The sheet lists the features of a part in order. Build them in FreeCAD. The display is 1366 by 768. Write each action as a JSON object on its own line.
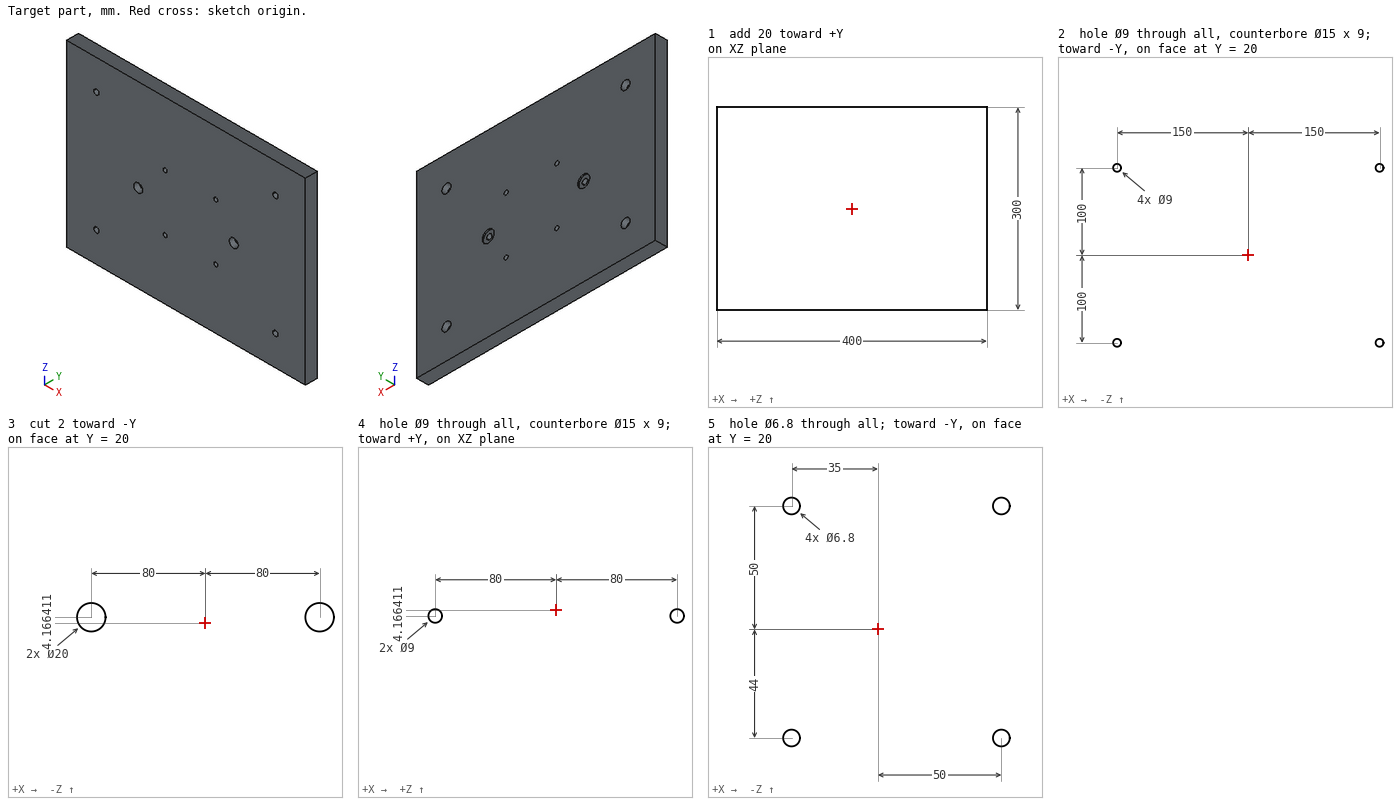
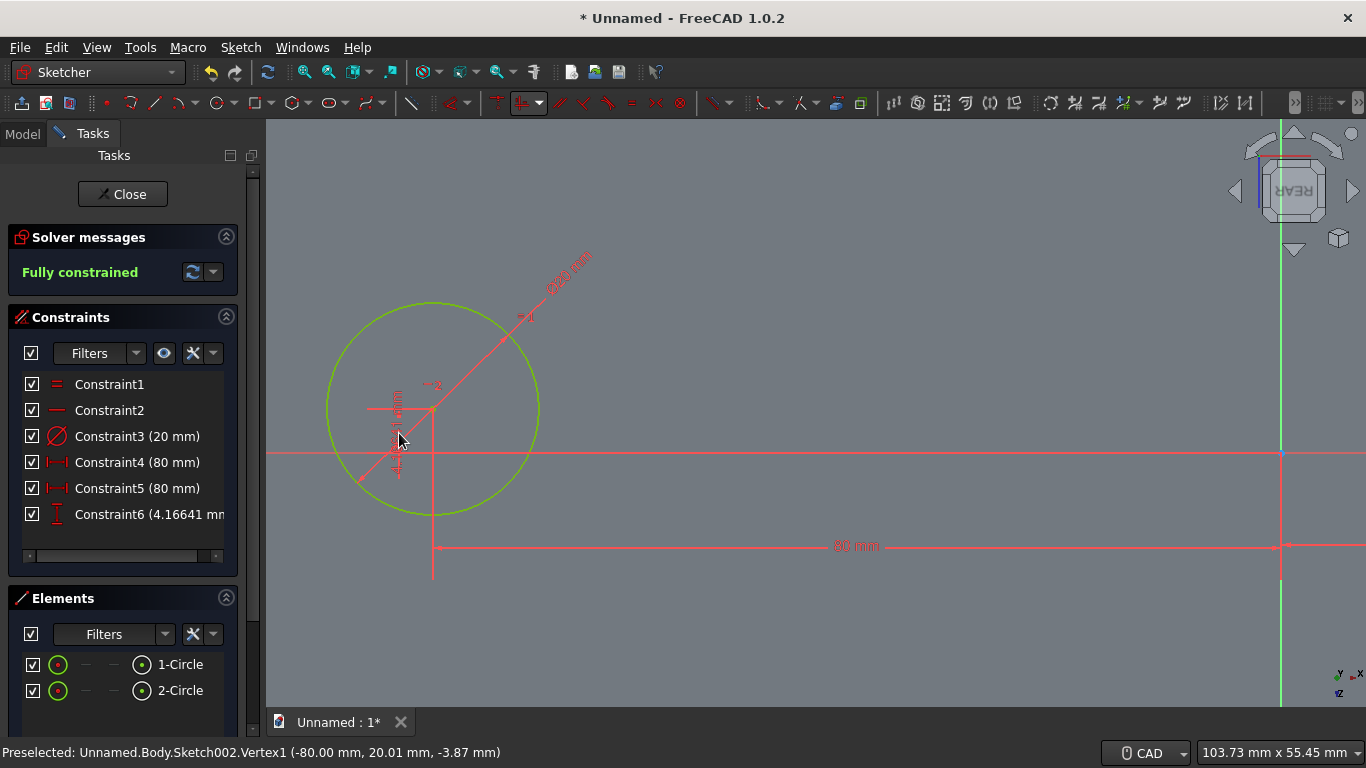
{"action": "left_click", "coordinate": [123, 194]}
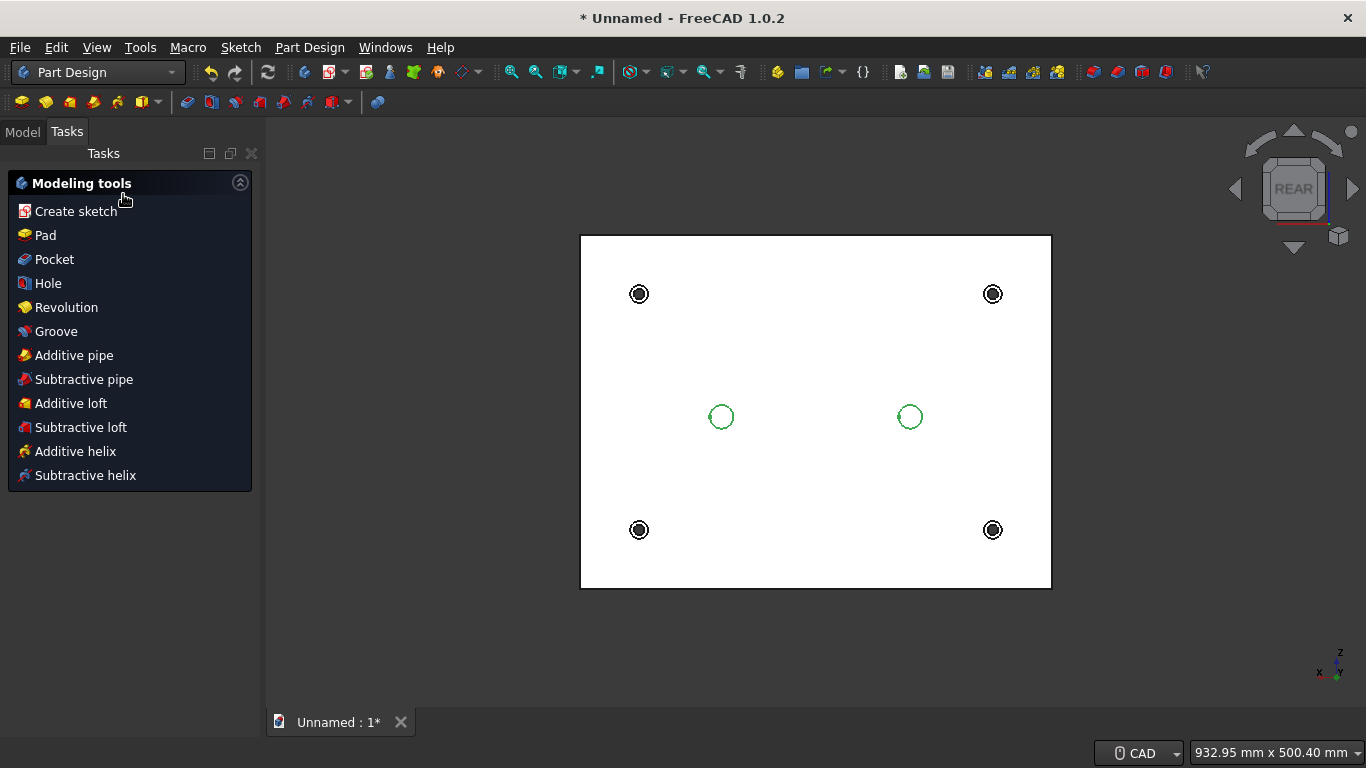
{"action": "left_click", "coordinate": [188, 102]}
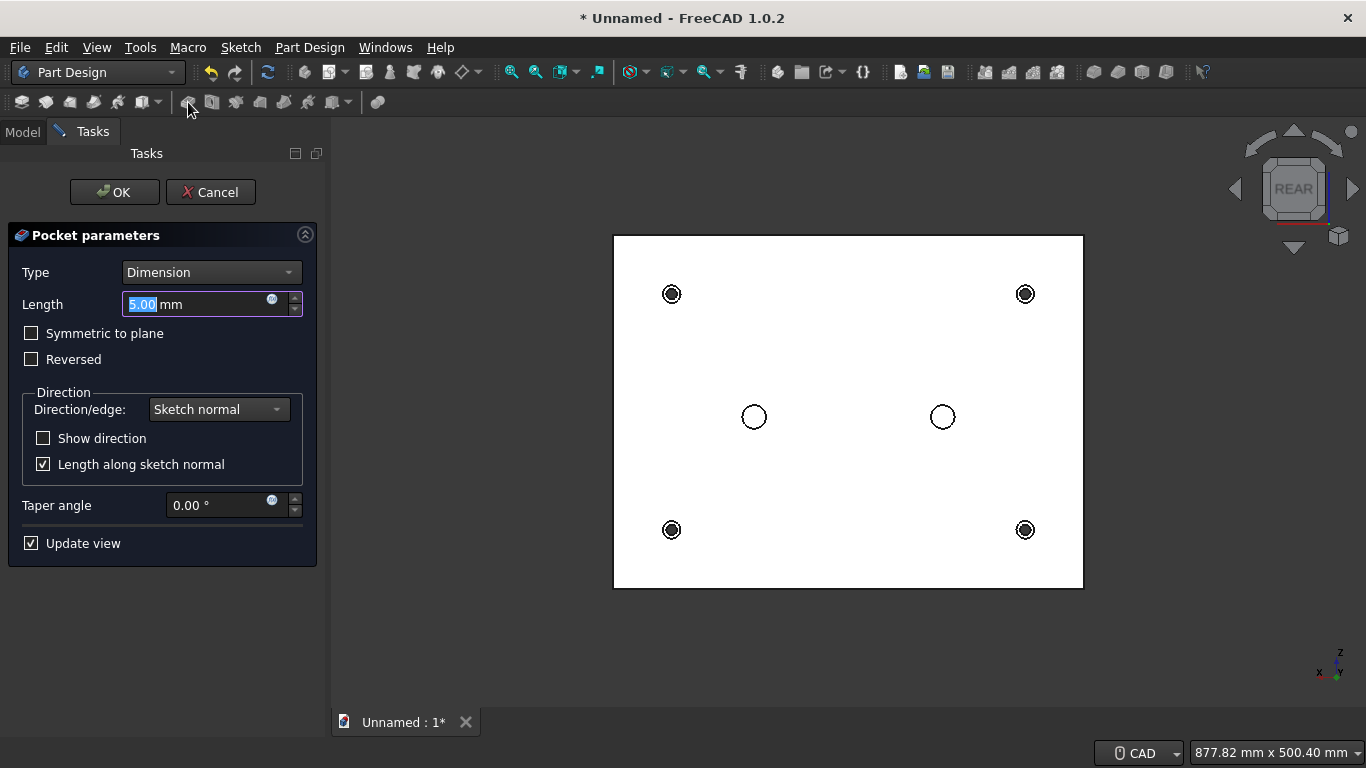
{"action": "type", "text": "2"}
{"action": "key", "text": "Tab"}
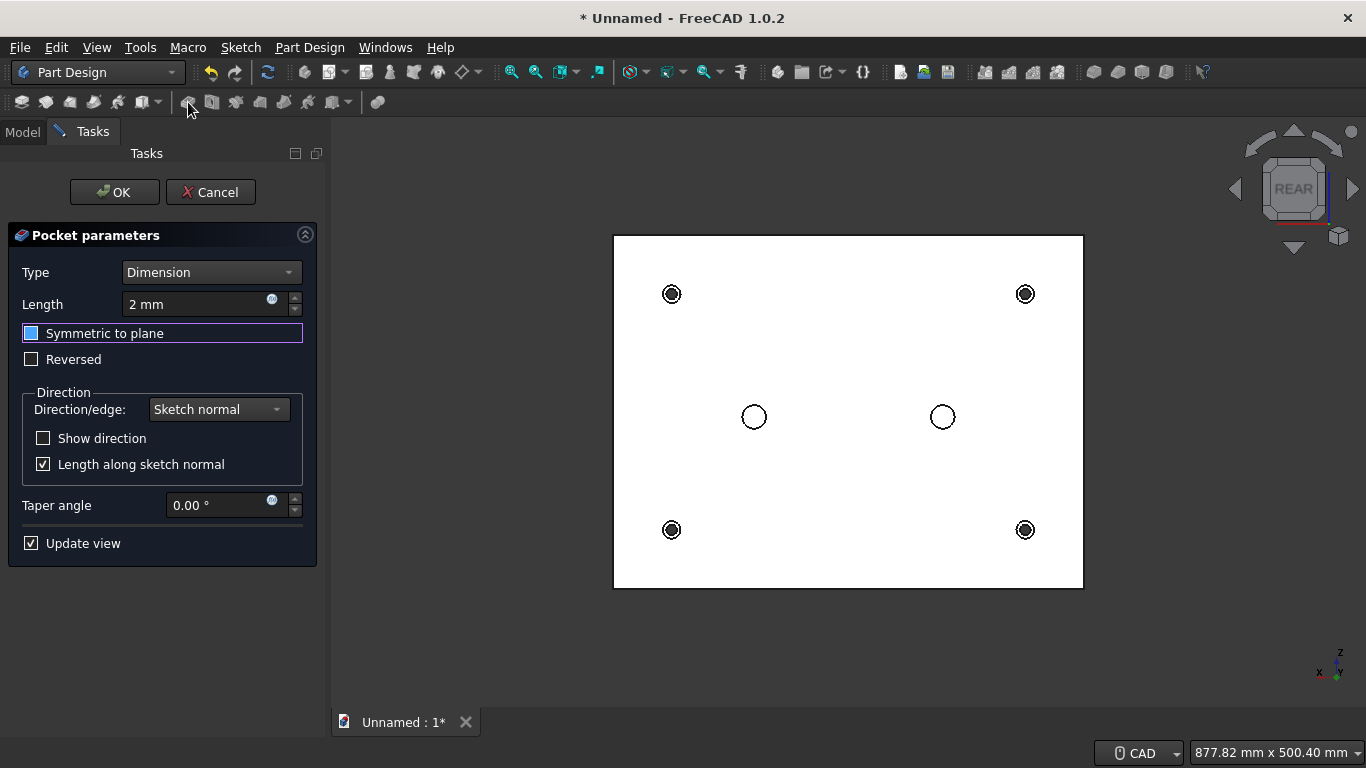
{"action": "left_click", "coordinate": [115, 192]}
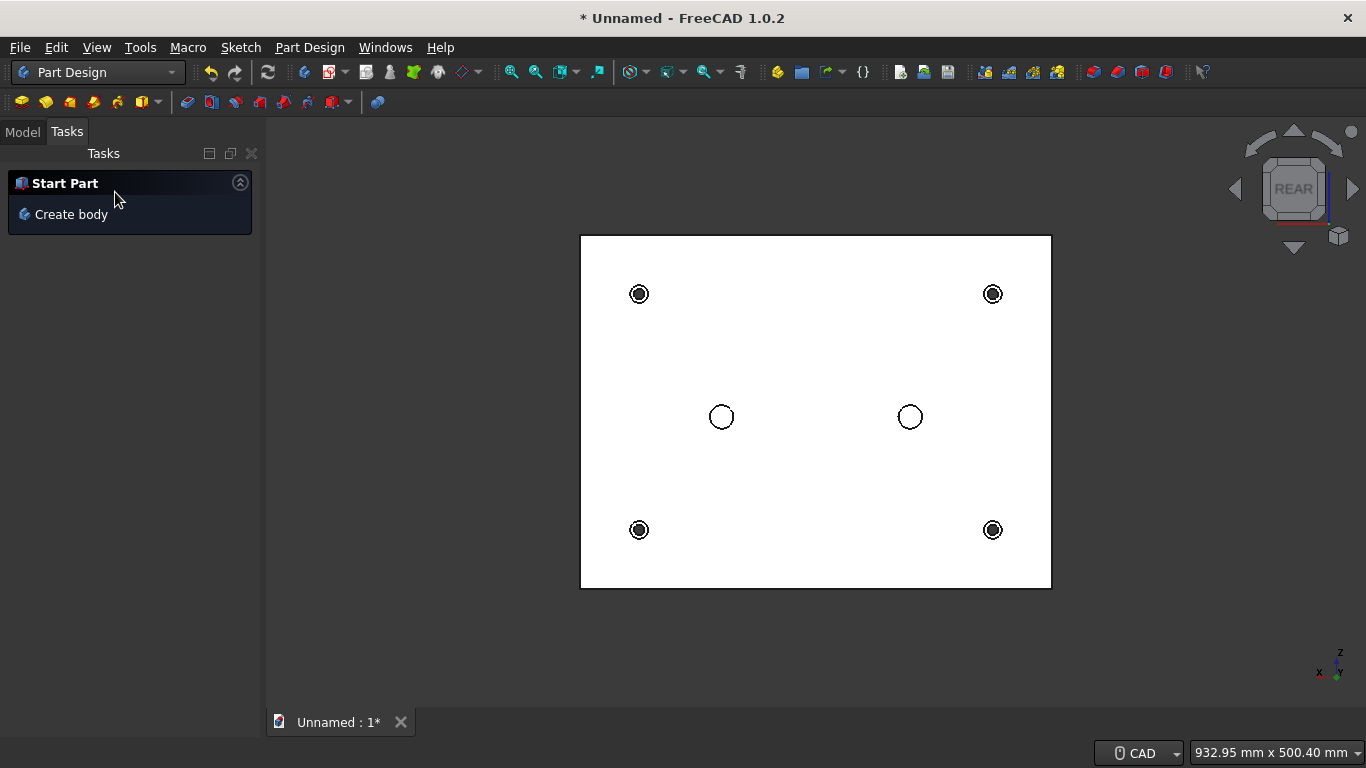
{"action": "left_click", "coordinate": [330, 72]}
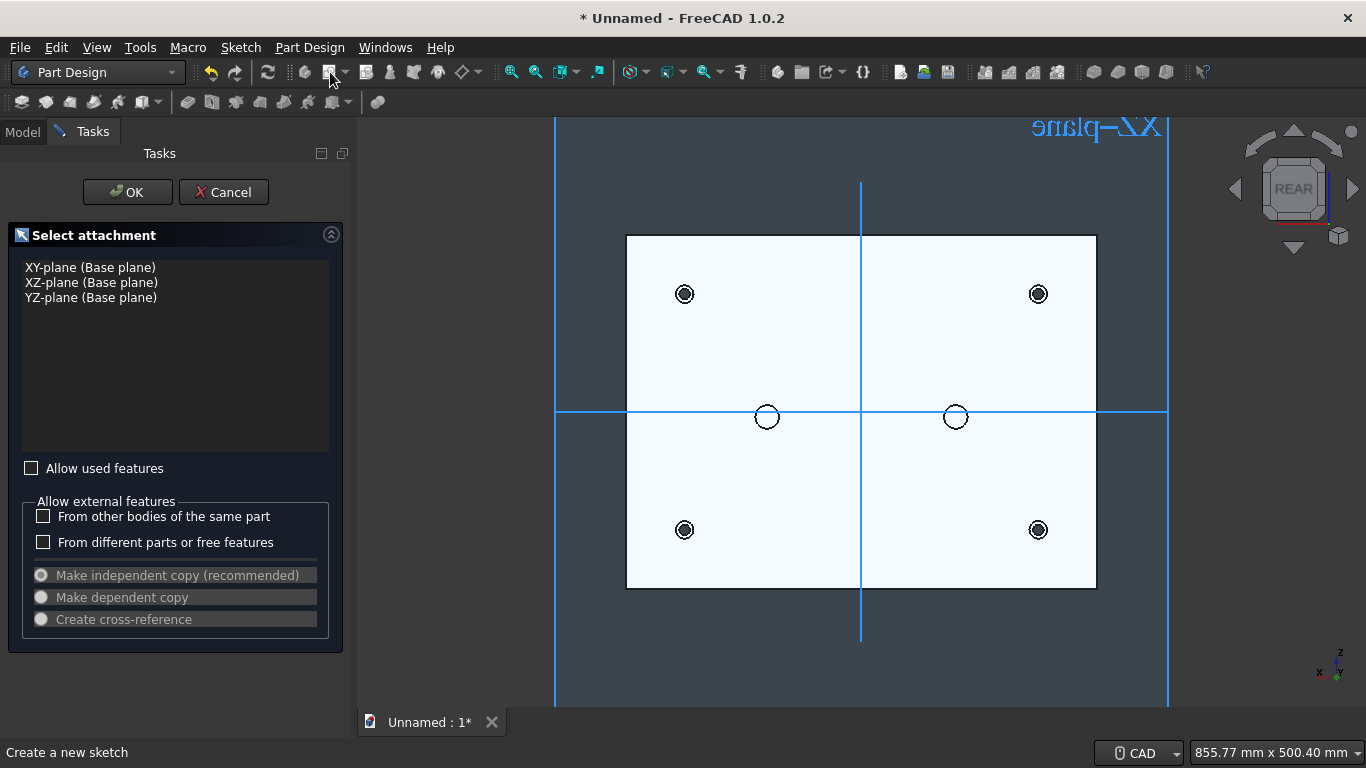
{"action": "left_click", "coordinate": [82, 282]}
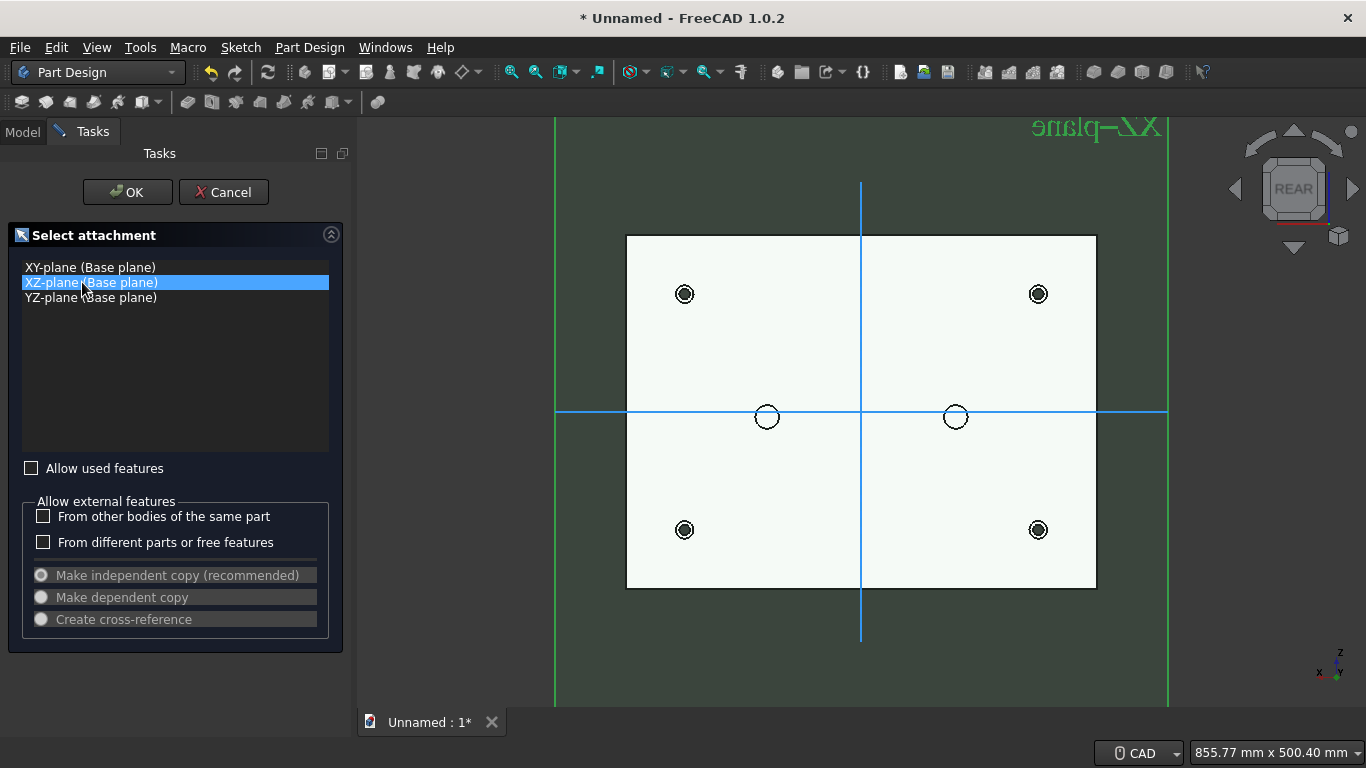
{"action": "left_click", "coordinate": [128, 192]}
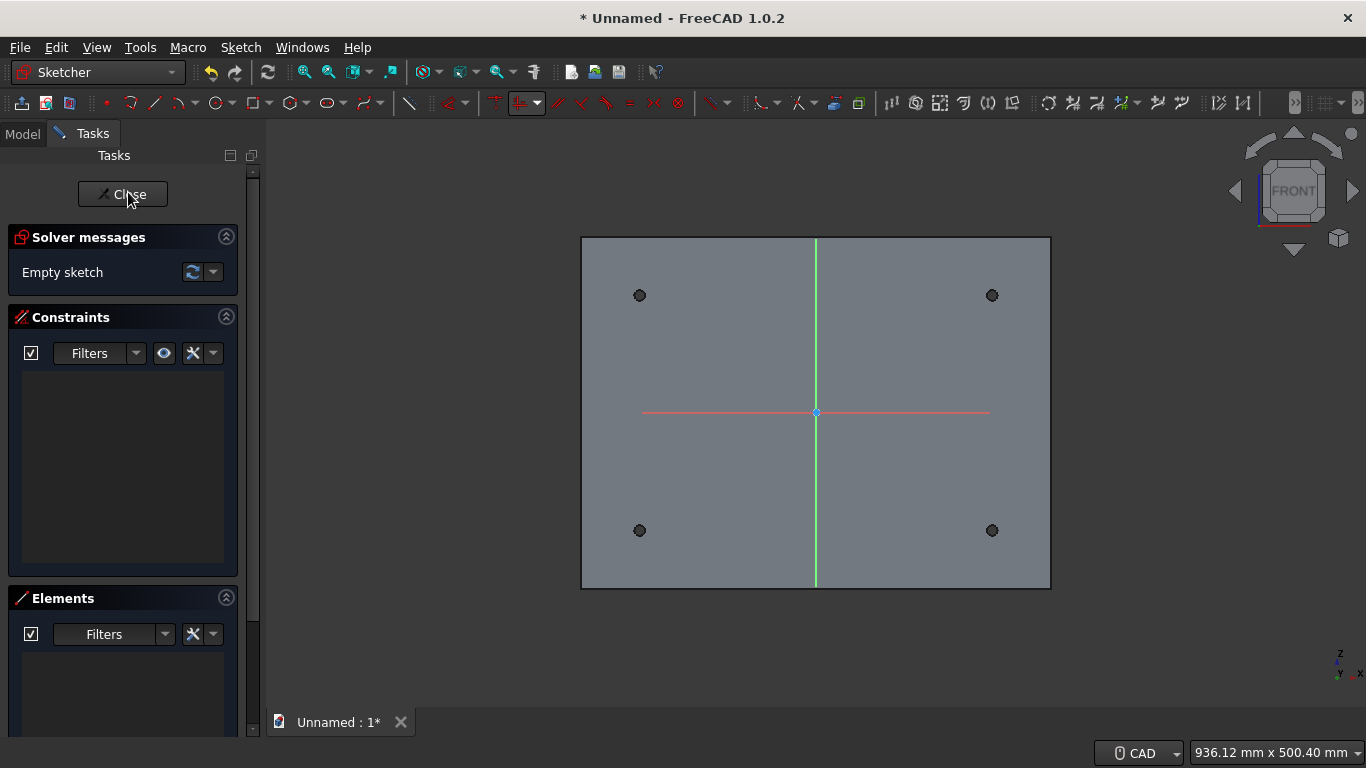
{"action": "scroll", "coordinate": [846, 420], "scroll_direction": "up", "scroll_amount": 6}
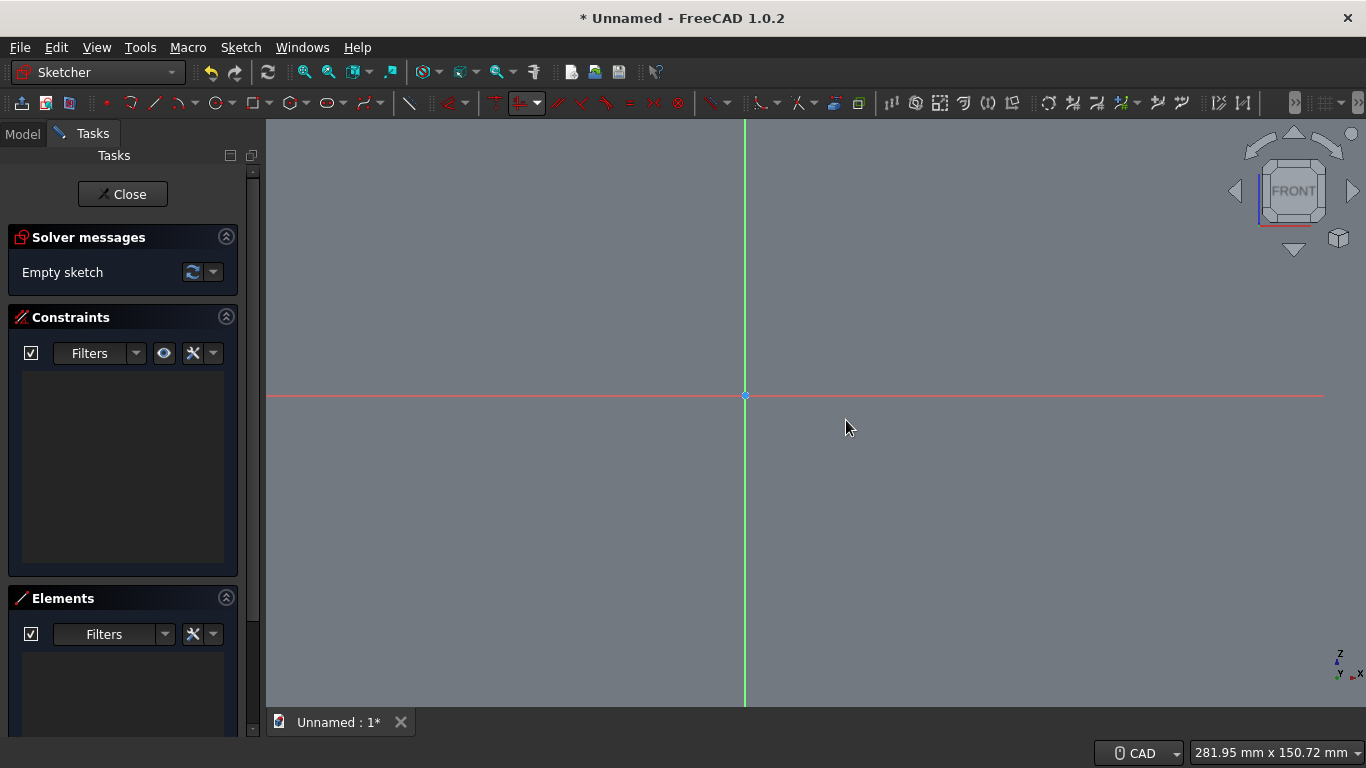
{"action": "key", "text": "g c"}